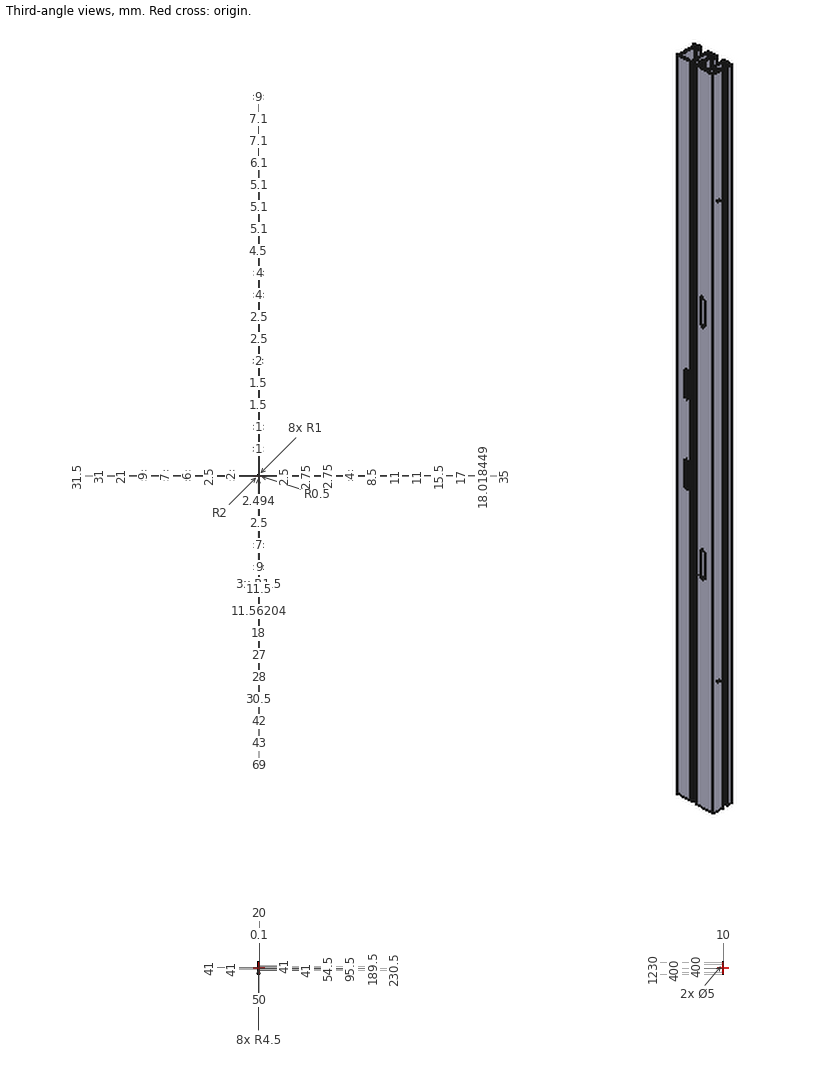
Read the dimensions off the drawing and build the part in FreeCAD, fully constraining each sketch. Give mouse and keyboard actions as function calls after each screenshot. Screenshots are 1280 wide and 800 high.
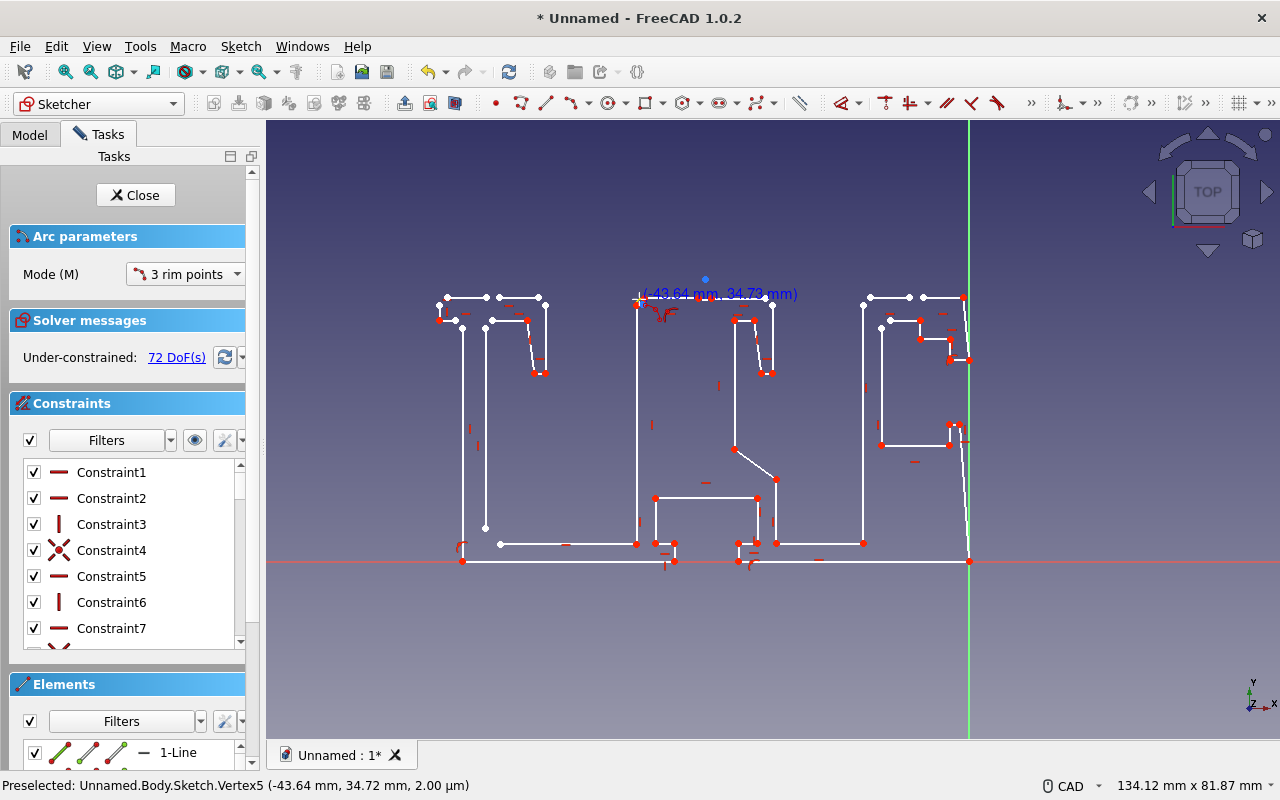
click(501, 544)
click(486, 529)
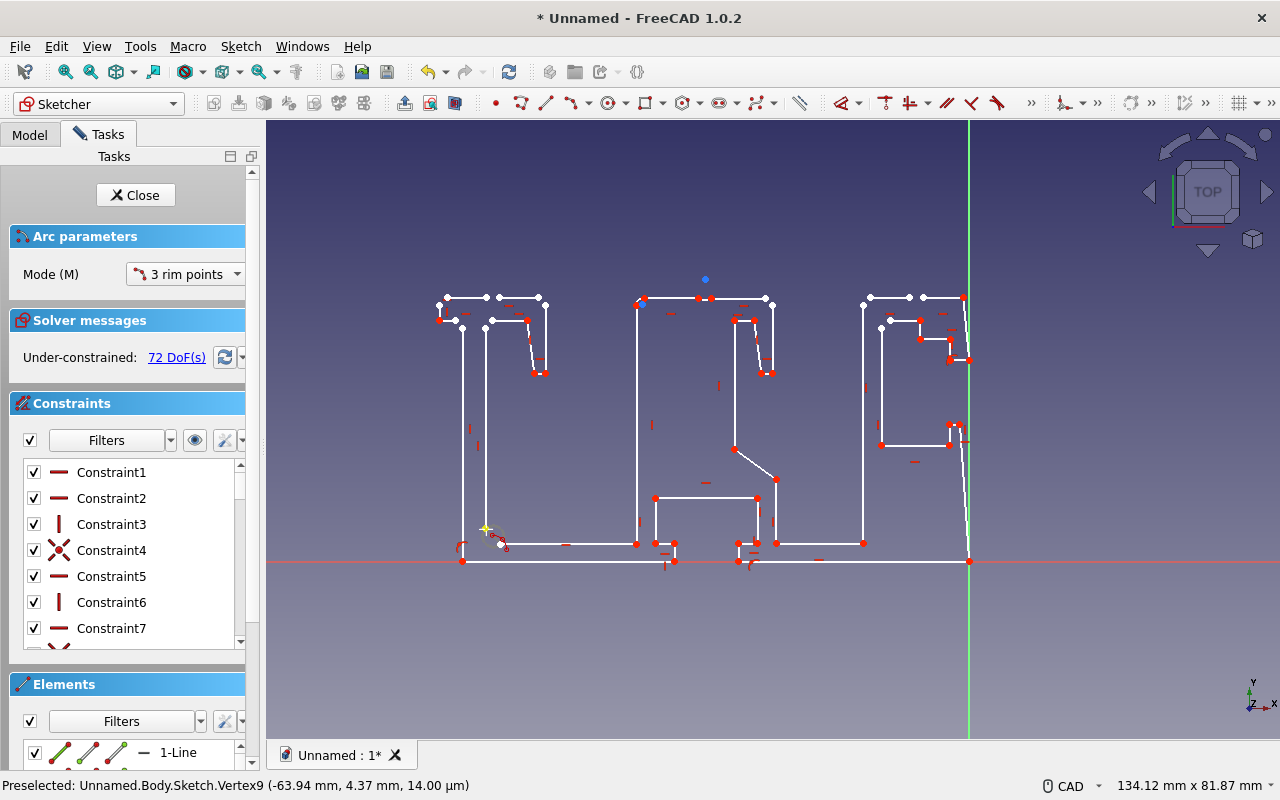
scroll(490, 539, up, 7)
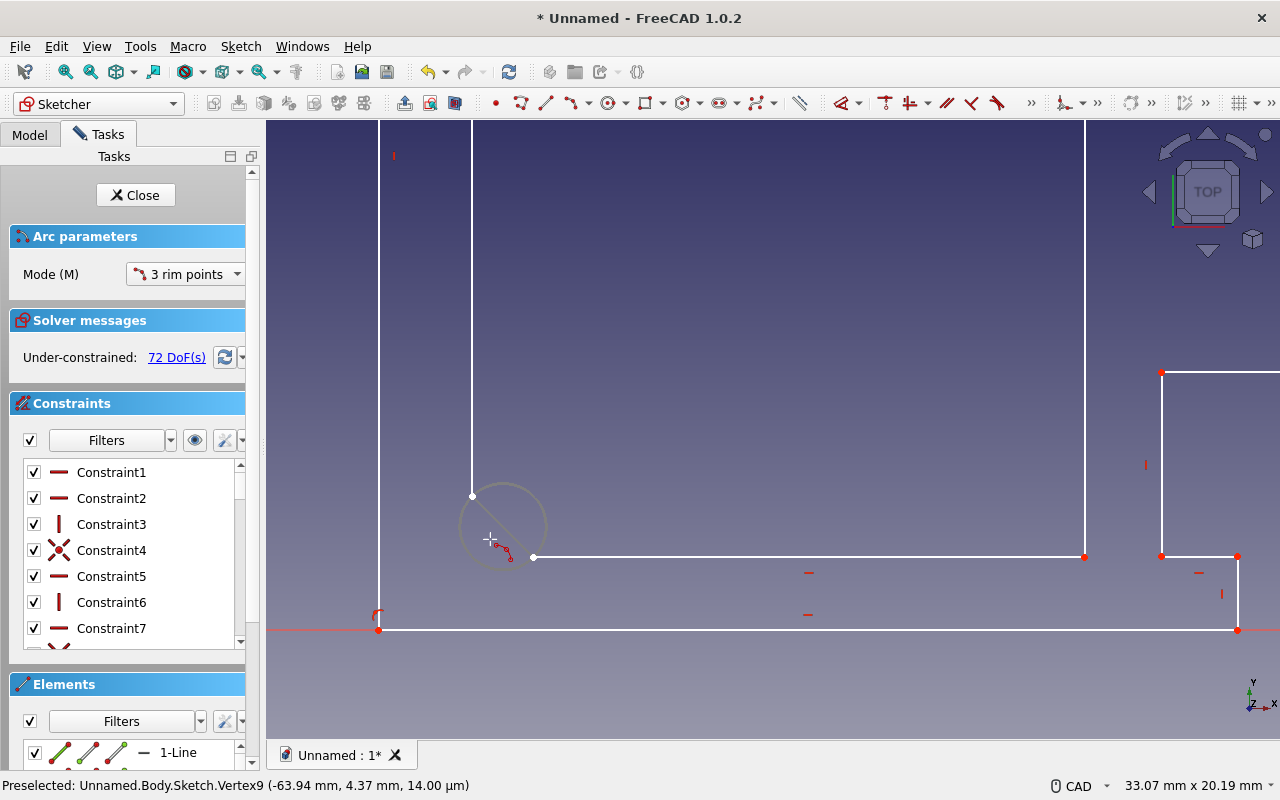
click(489, 535)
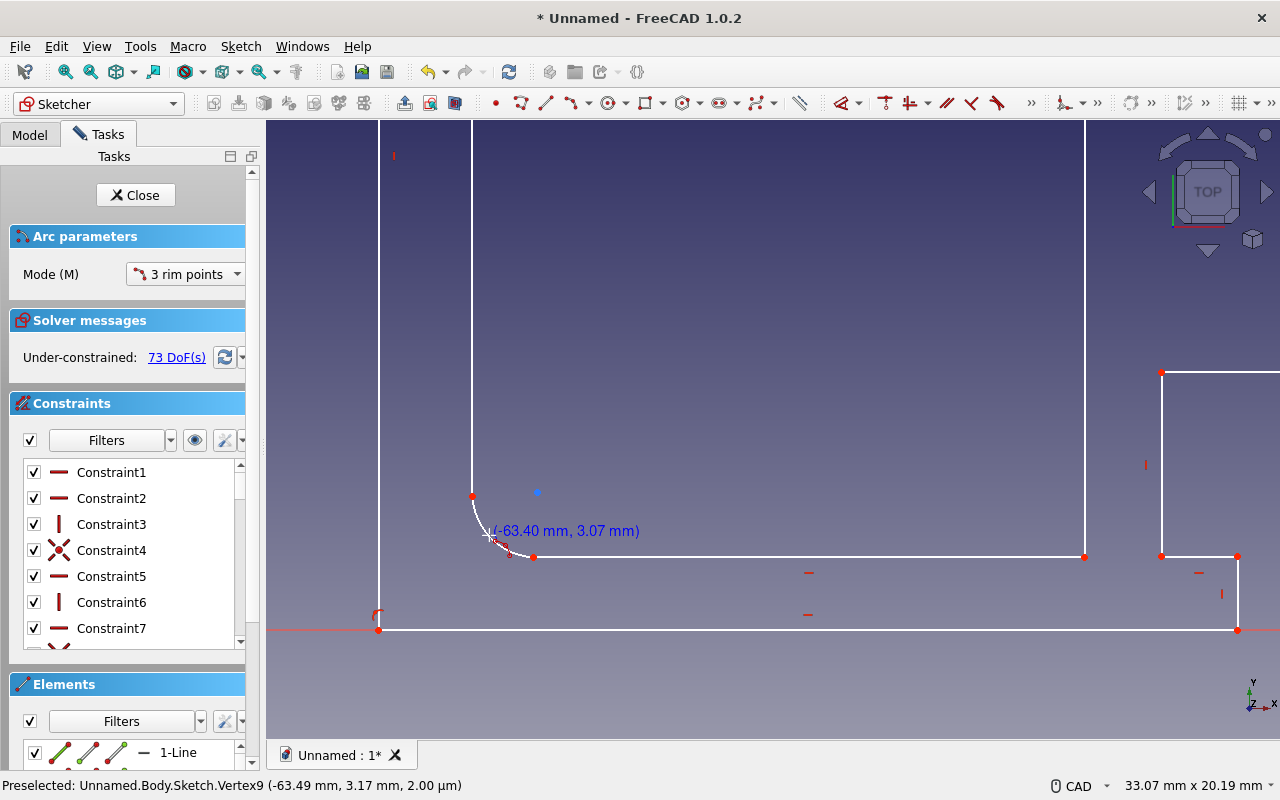
scroll(490, 539, down, 7)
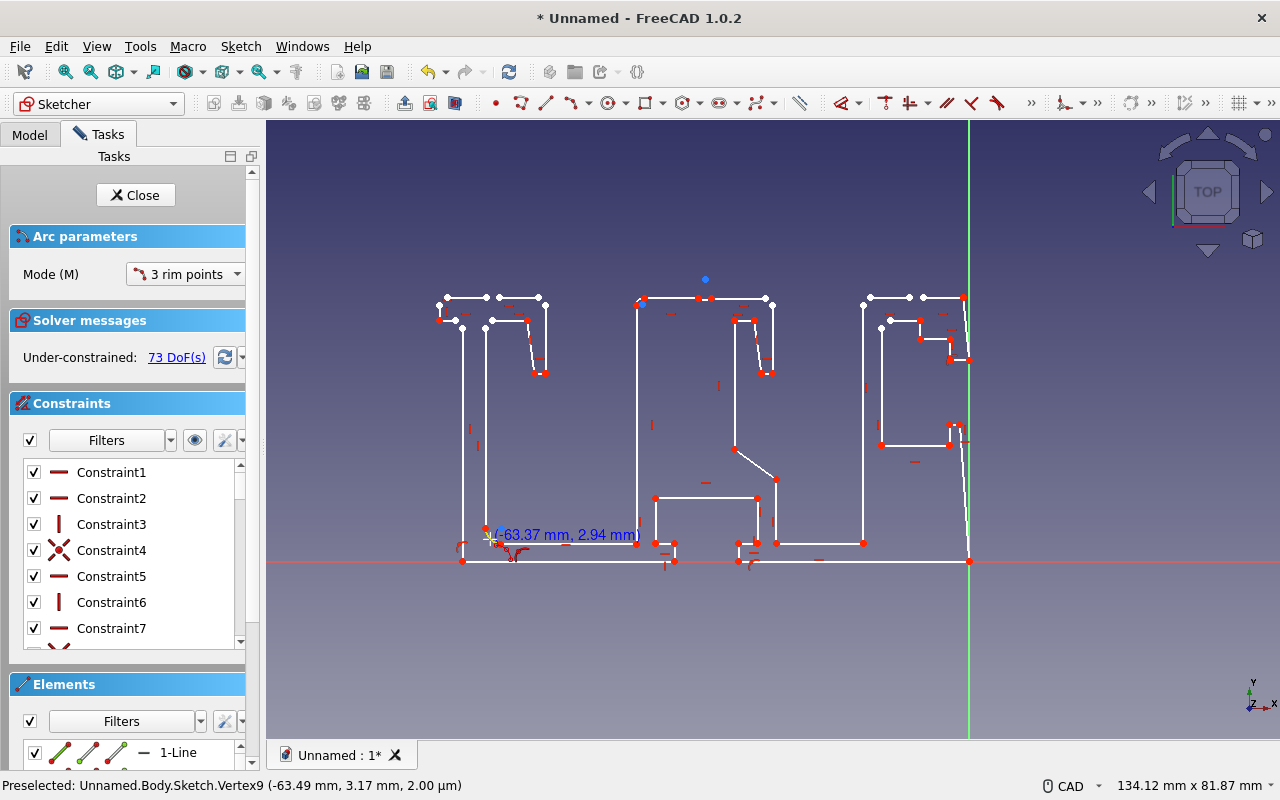
scroll(485, 328, up, 2)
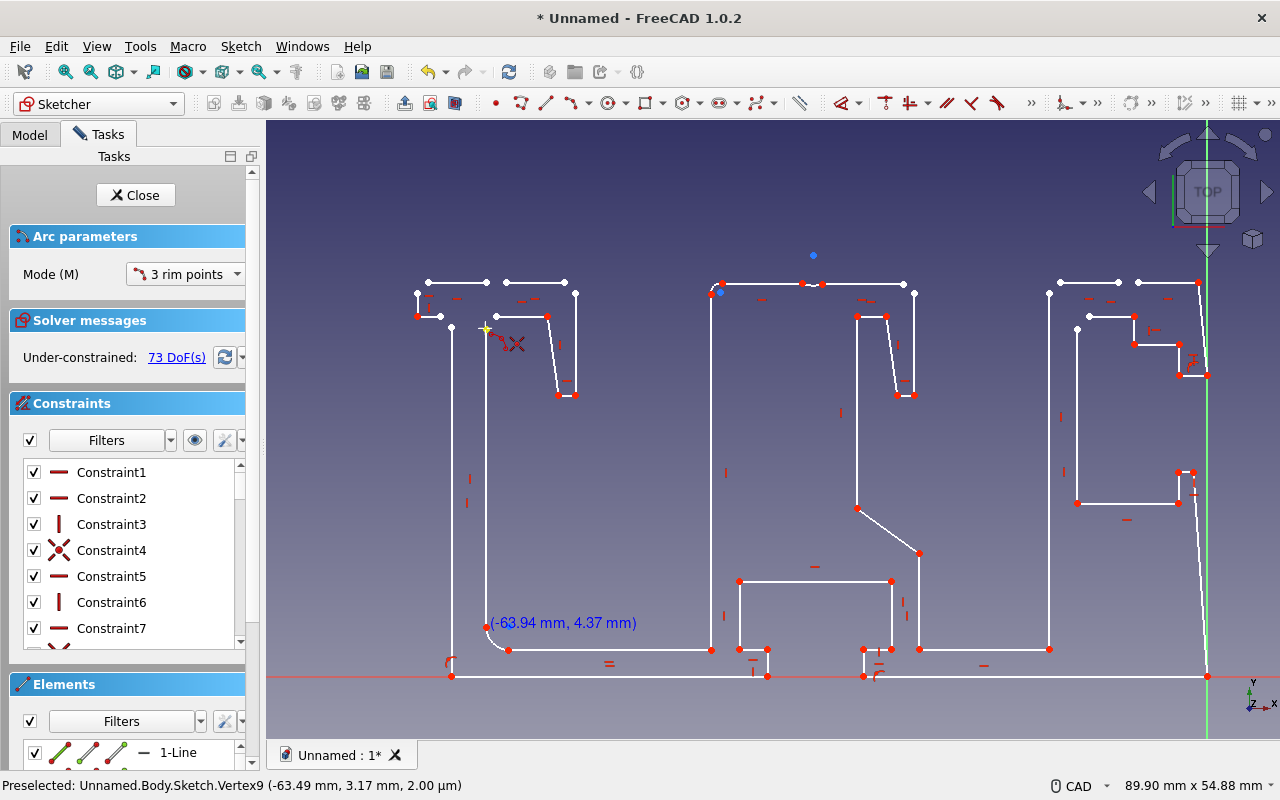
click(486, 329)
click(497, 317)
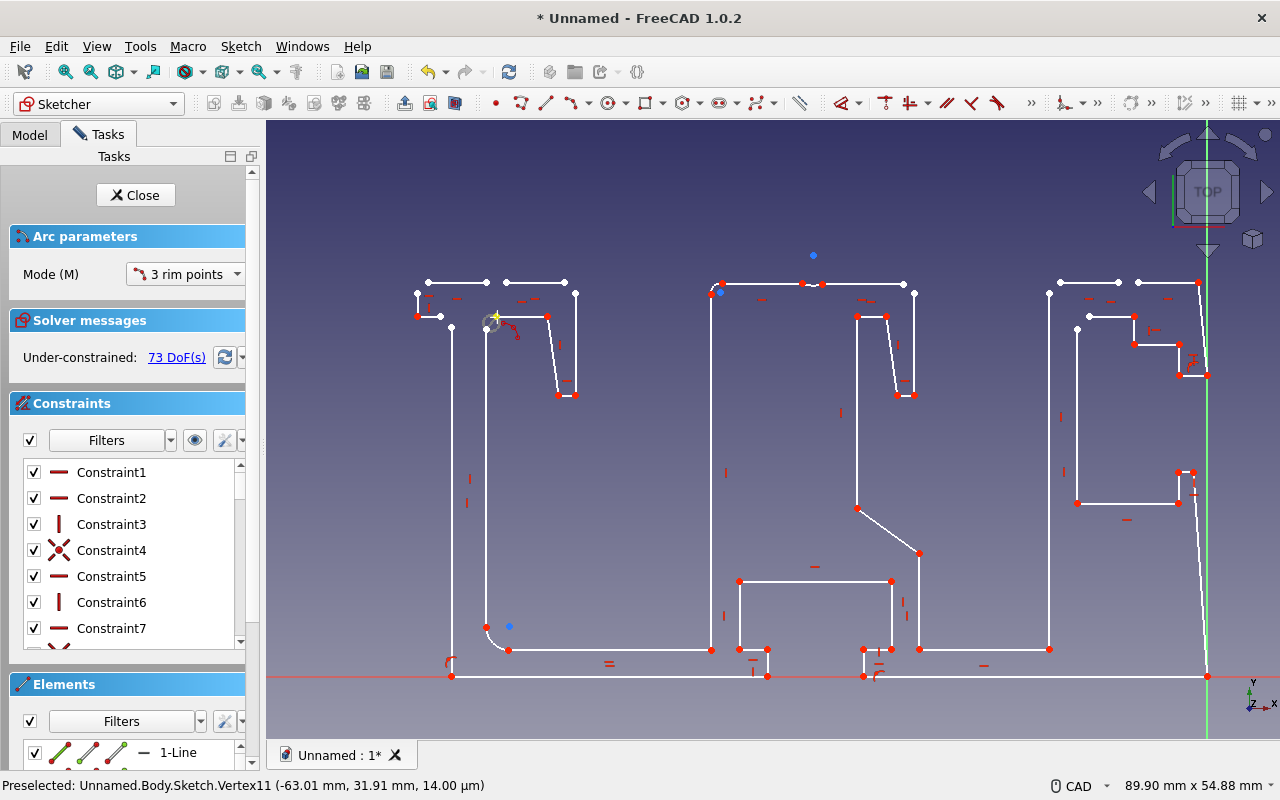
scroll(489, 319, up, 8)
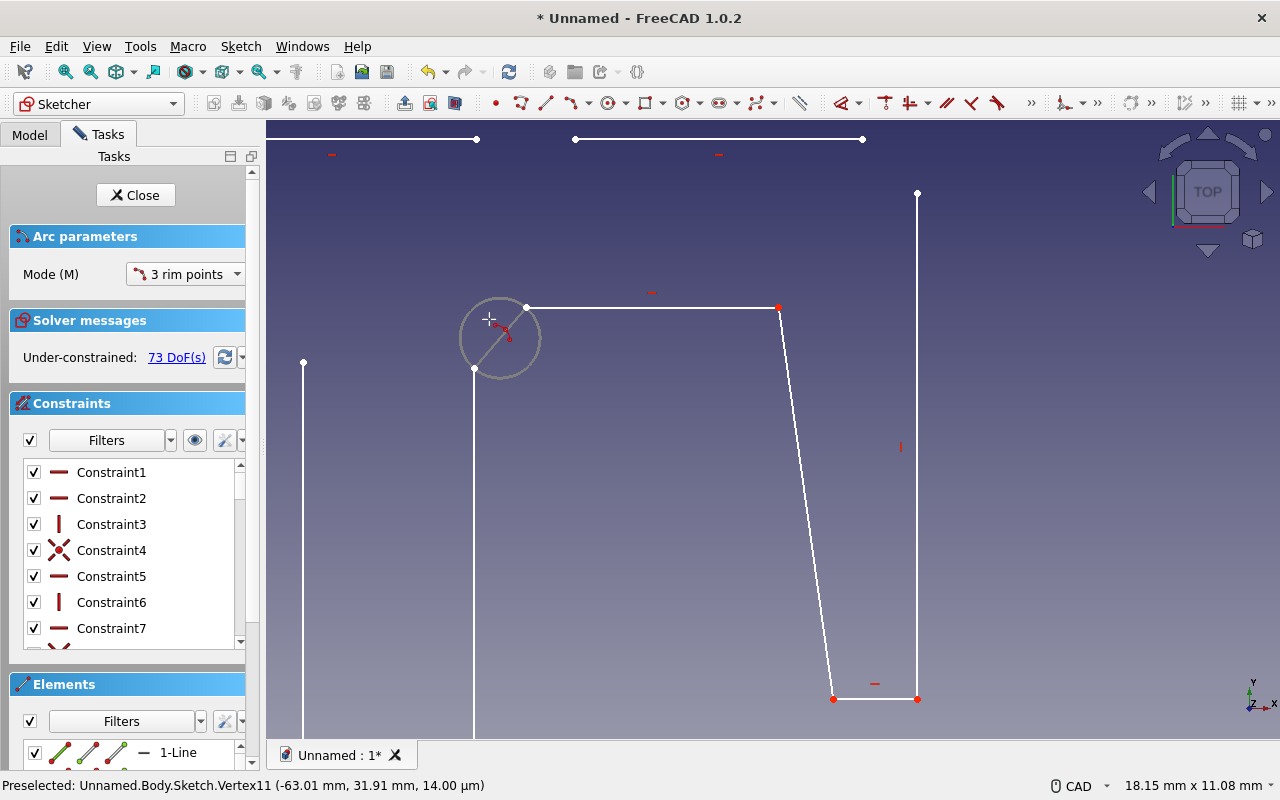
click(487, 319)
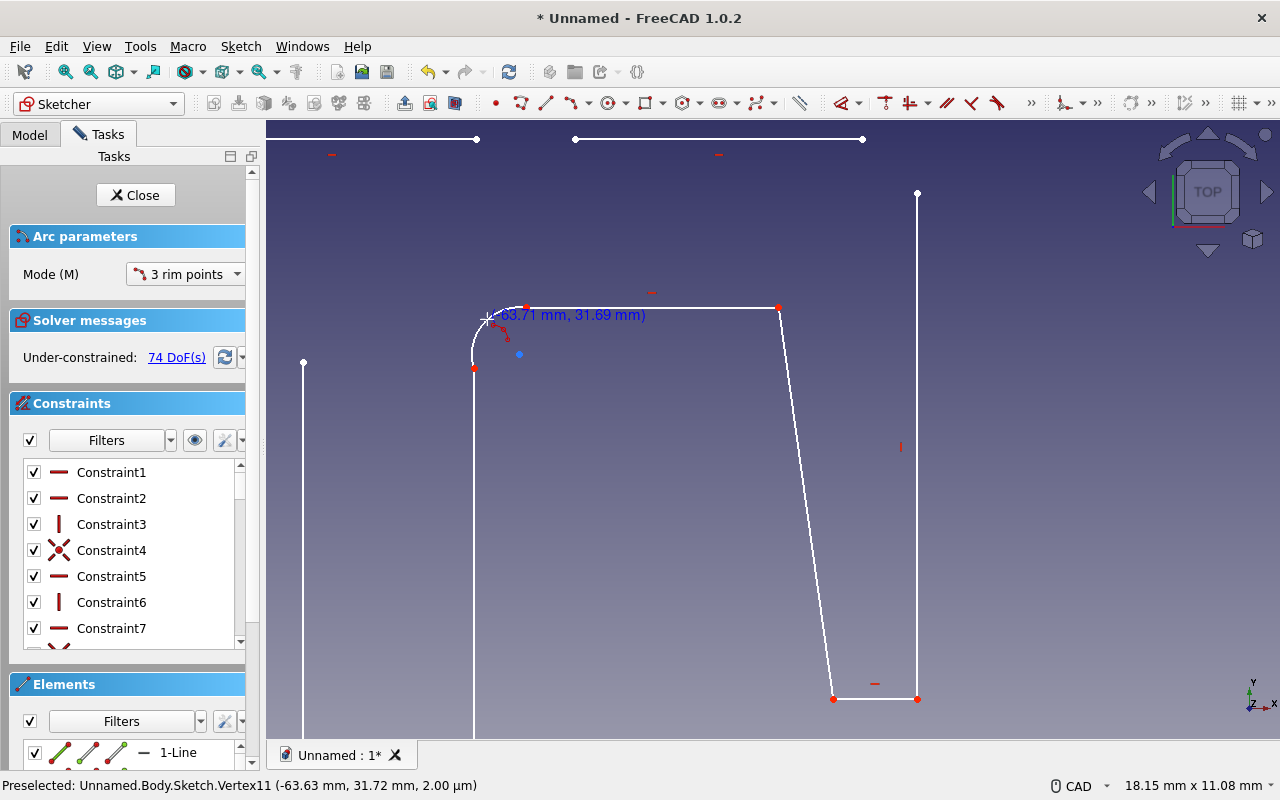
scroll(488, 323, down, 10)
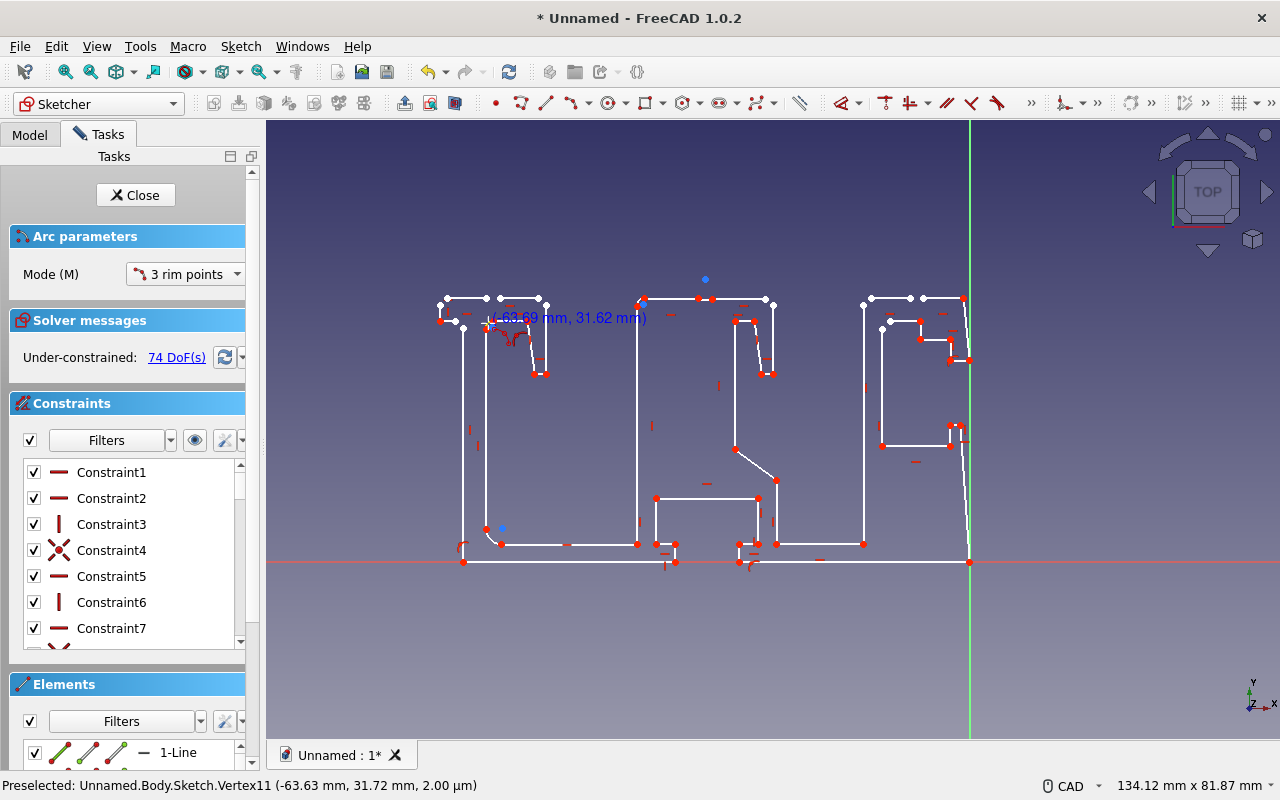
scroll(546, 305, up, 2)